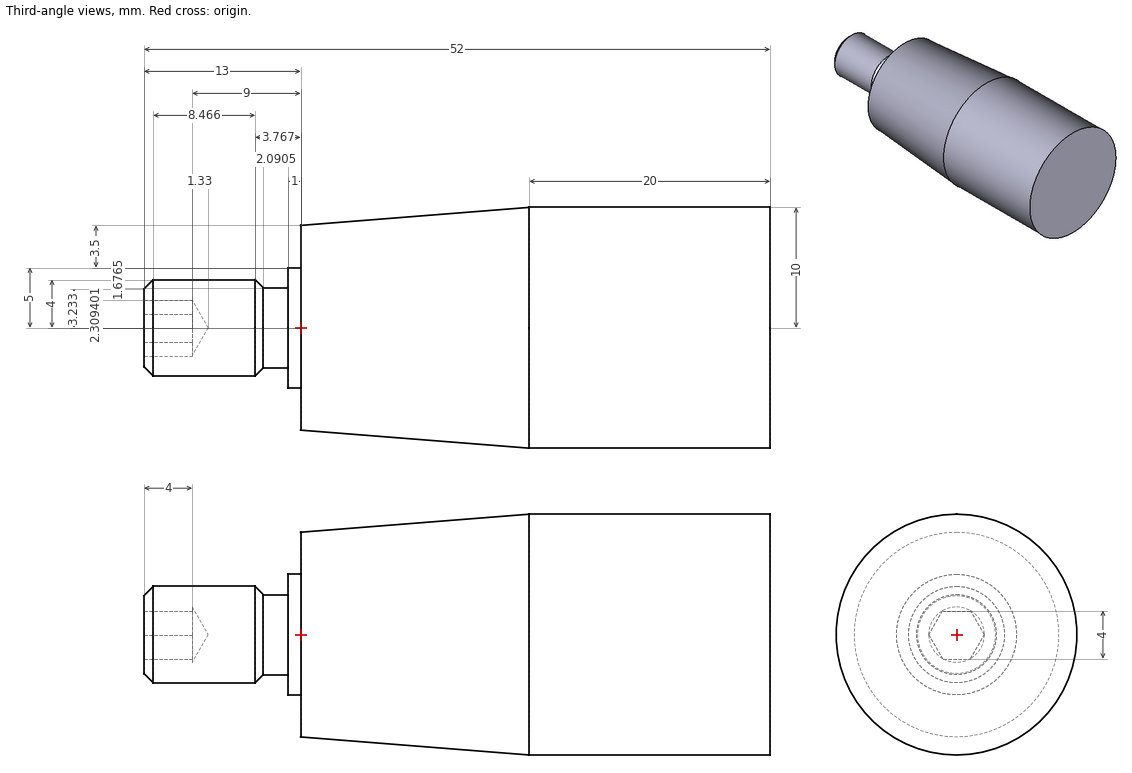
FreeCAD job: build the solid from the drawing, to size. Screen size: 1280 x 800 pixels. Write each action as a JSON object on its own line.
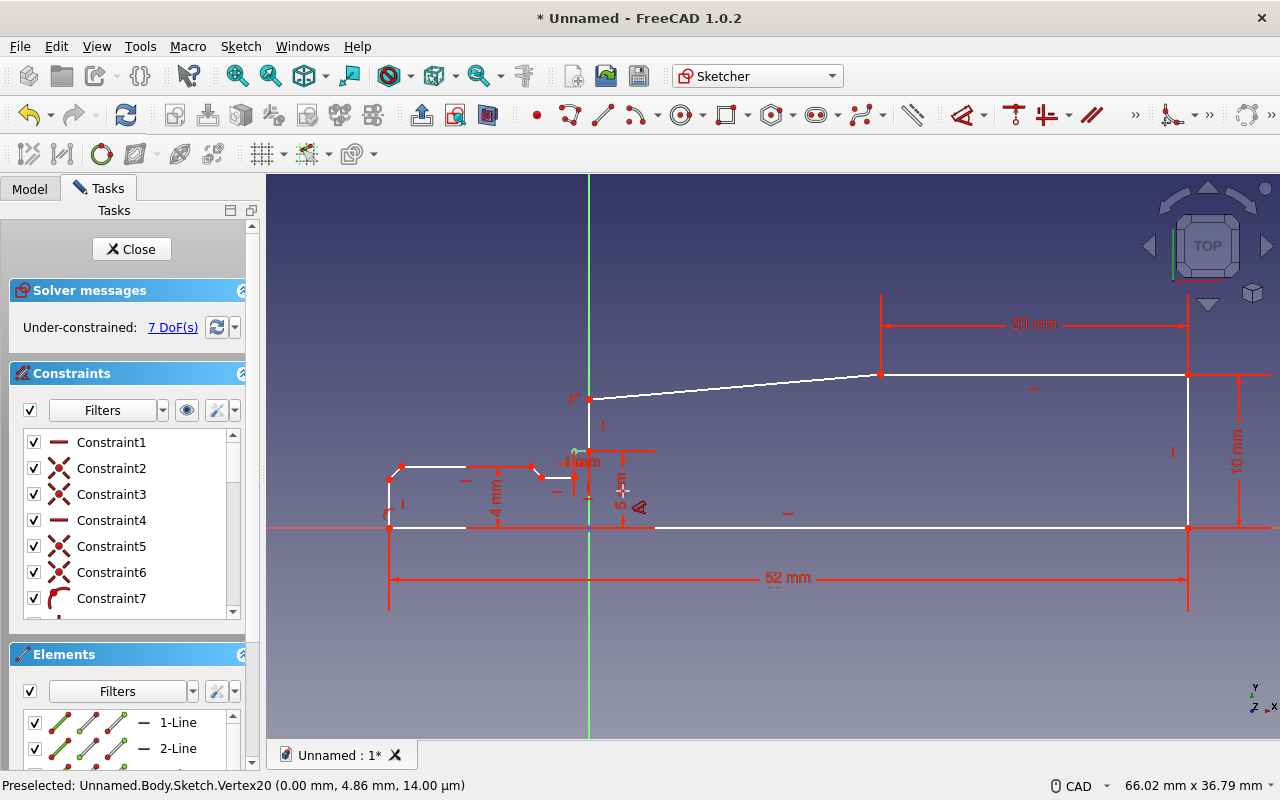
{"action": "left_click", "coordinate": [589, 415]}
{"action": "left_click", "coordinate": [555, 426]}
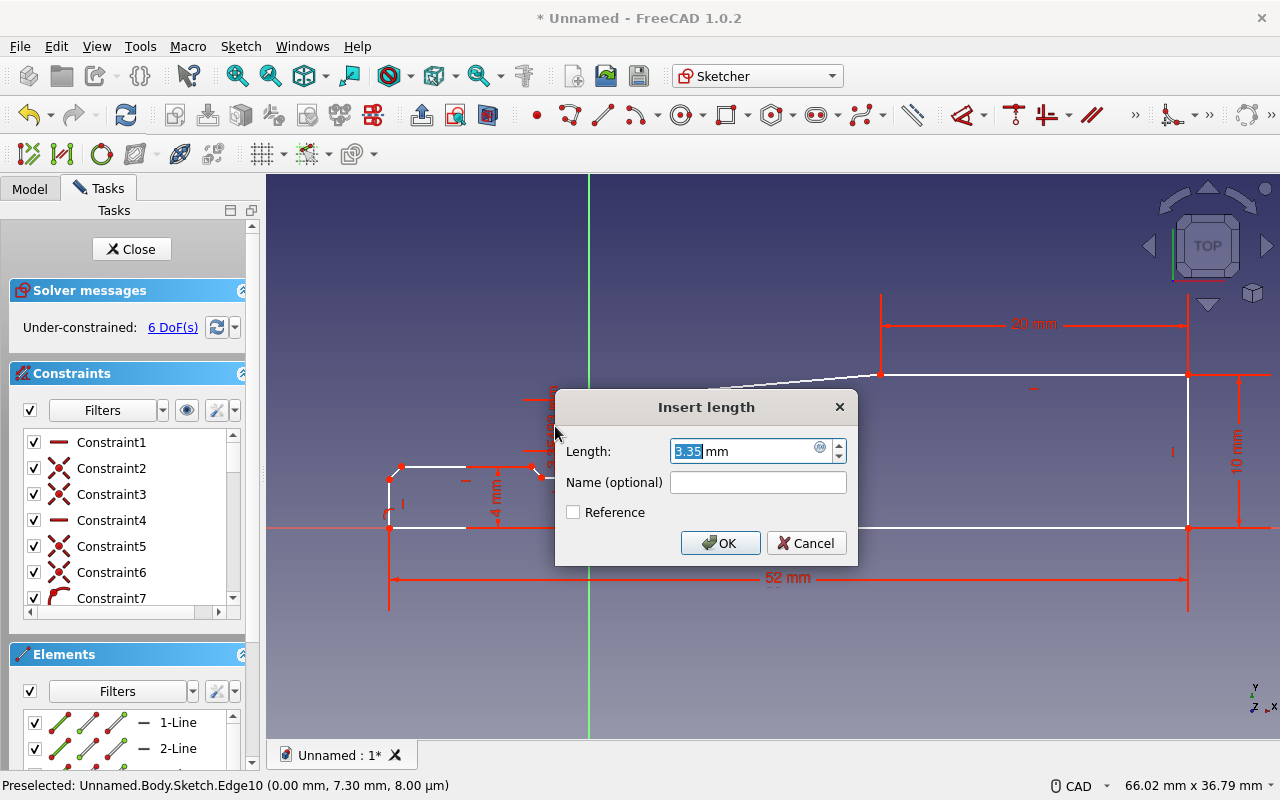
{"action": "type", "text": "3.5"}
{"action": "key", "text": "Return"}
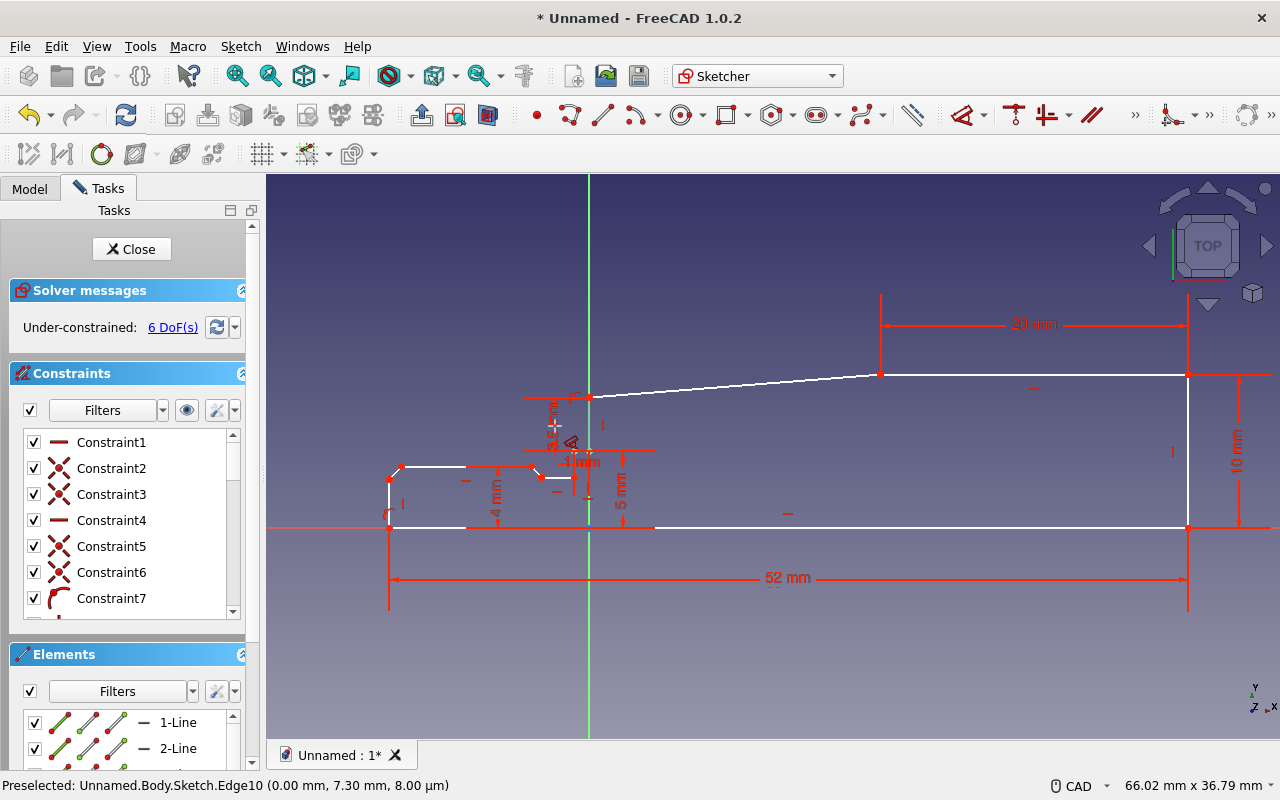
{"action": "left_click", "coordinate": [389, 479]}
{"action": "left_click", "coordinate": [489, 562]}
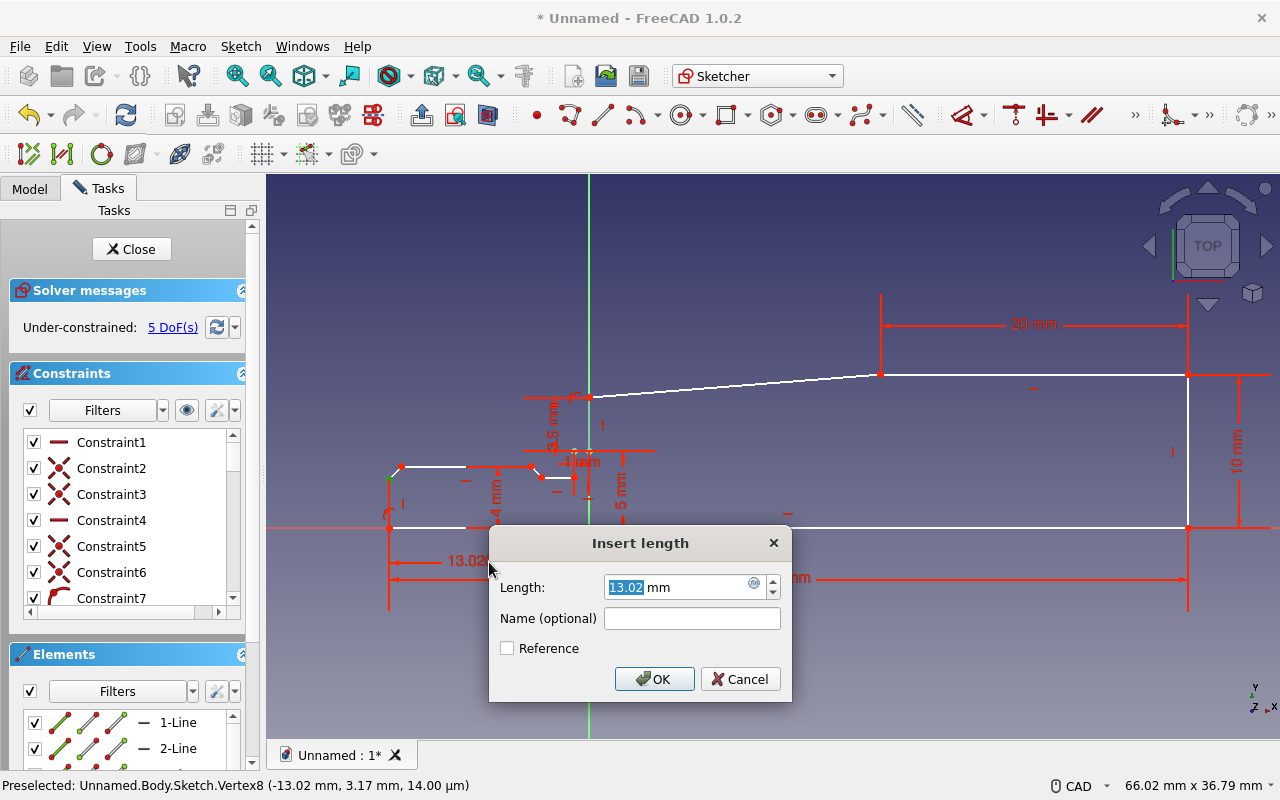
{"action": "type", "text": "13"}
{"action": "key", "text": "Return"}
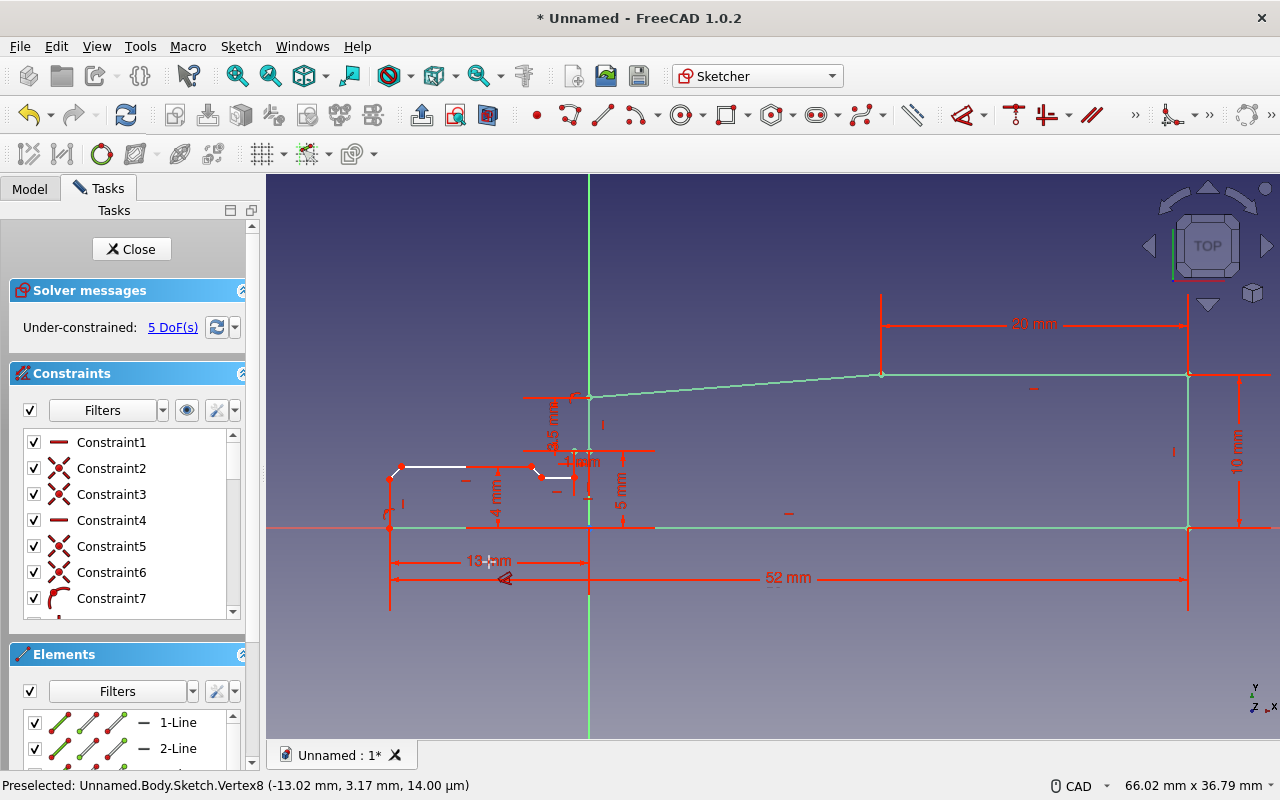
{"action": "left_click", "coordinate": [493, 467]}
{"action": "left_click", "coordinate": [421, 501]}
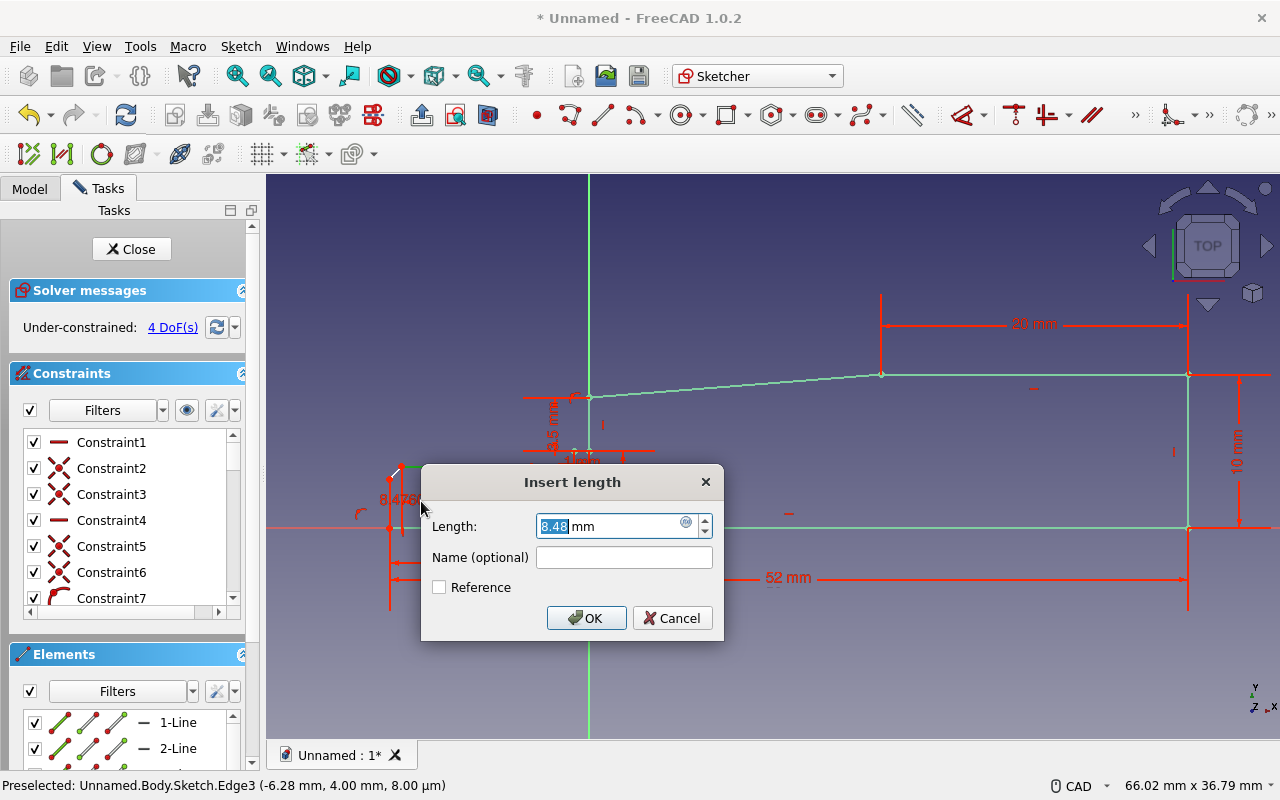
{"action": "type", "text": "8.466"}
{"action": "key", "text": "Return"}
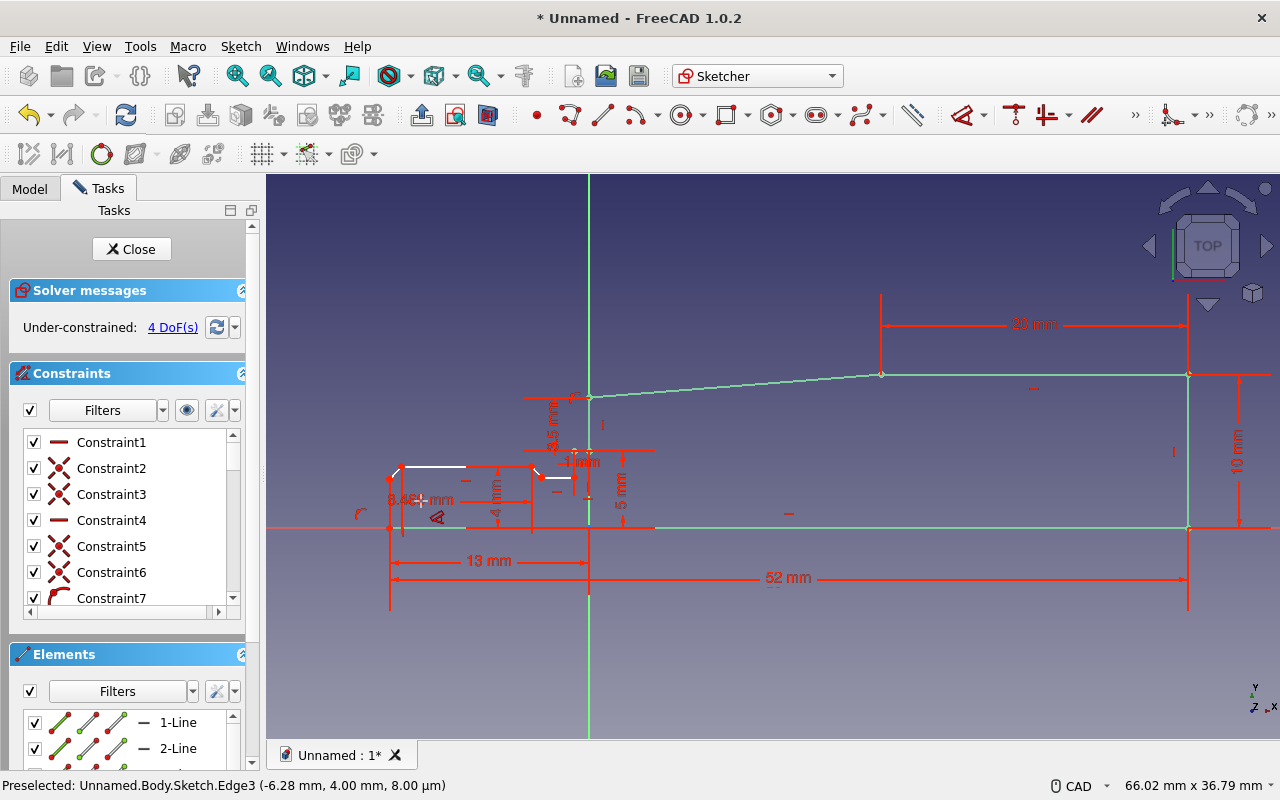
{"action": "left_click", "coordinate": [390, 494]}
{"action": "left_click", "coordinate": [332, 504]}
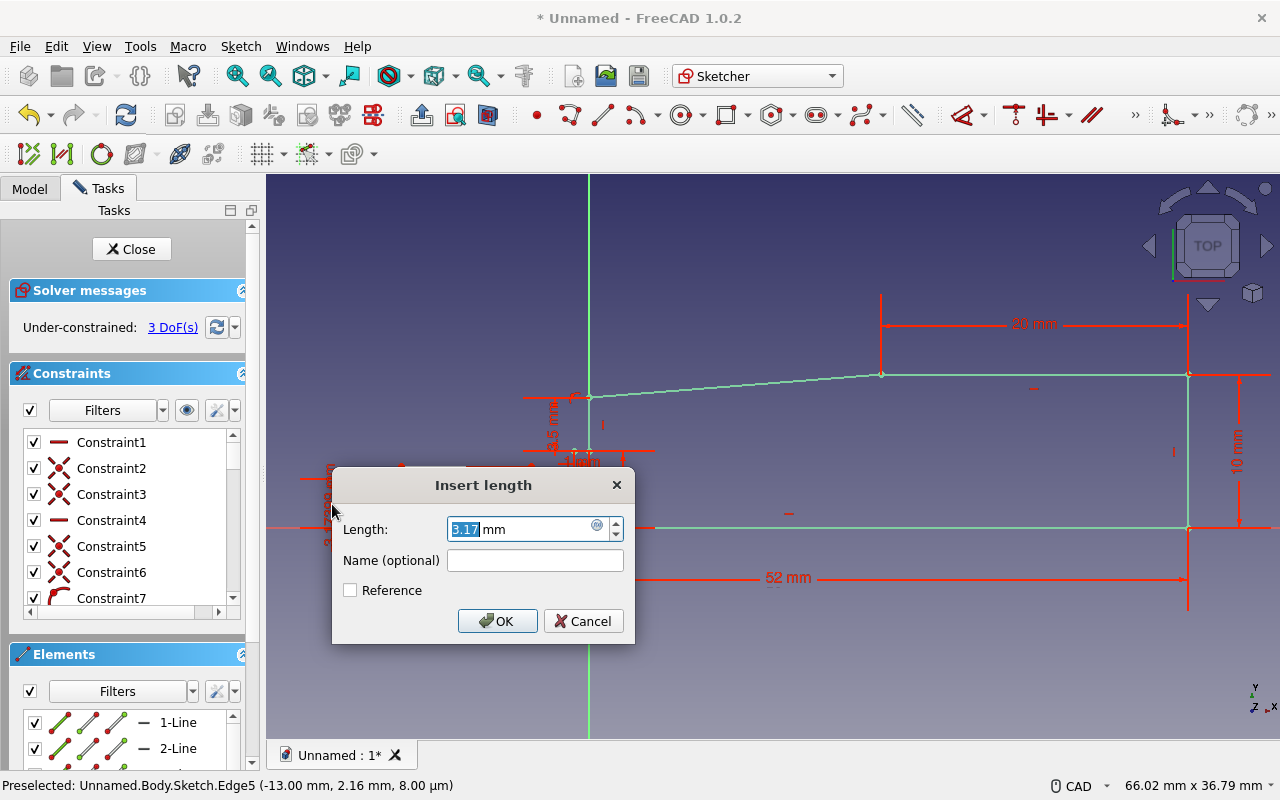
{"action": "type", "text": "3.233"}
{"action": "key", "text": "Return"}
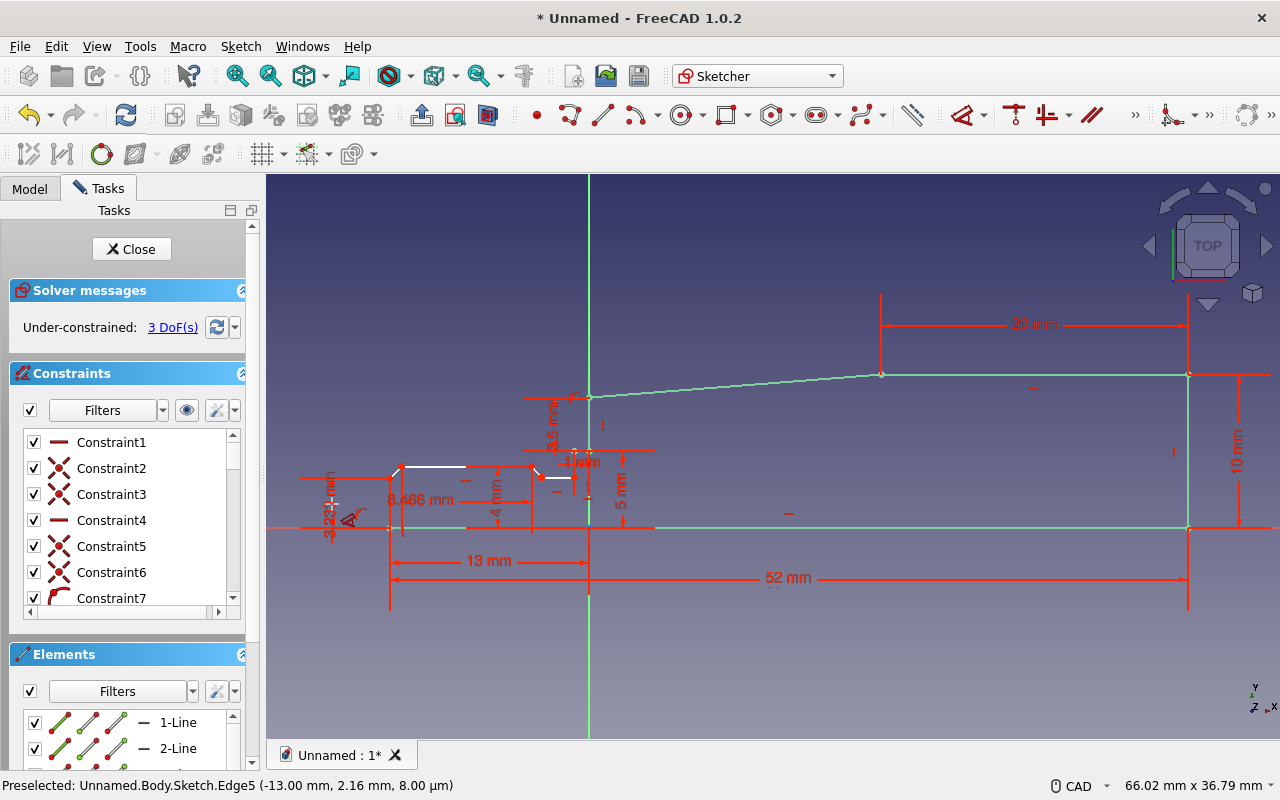
{"action": "scroll", "coordinate": [564, 478], "scroll_direction": "up", "scroll_amount": 2}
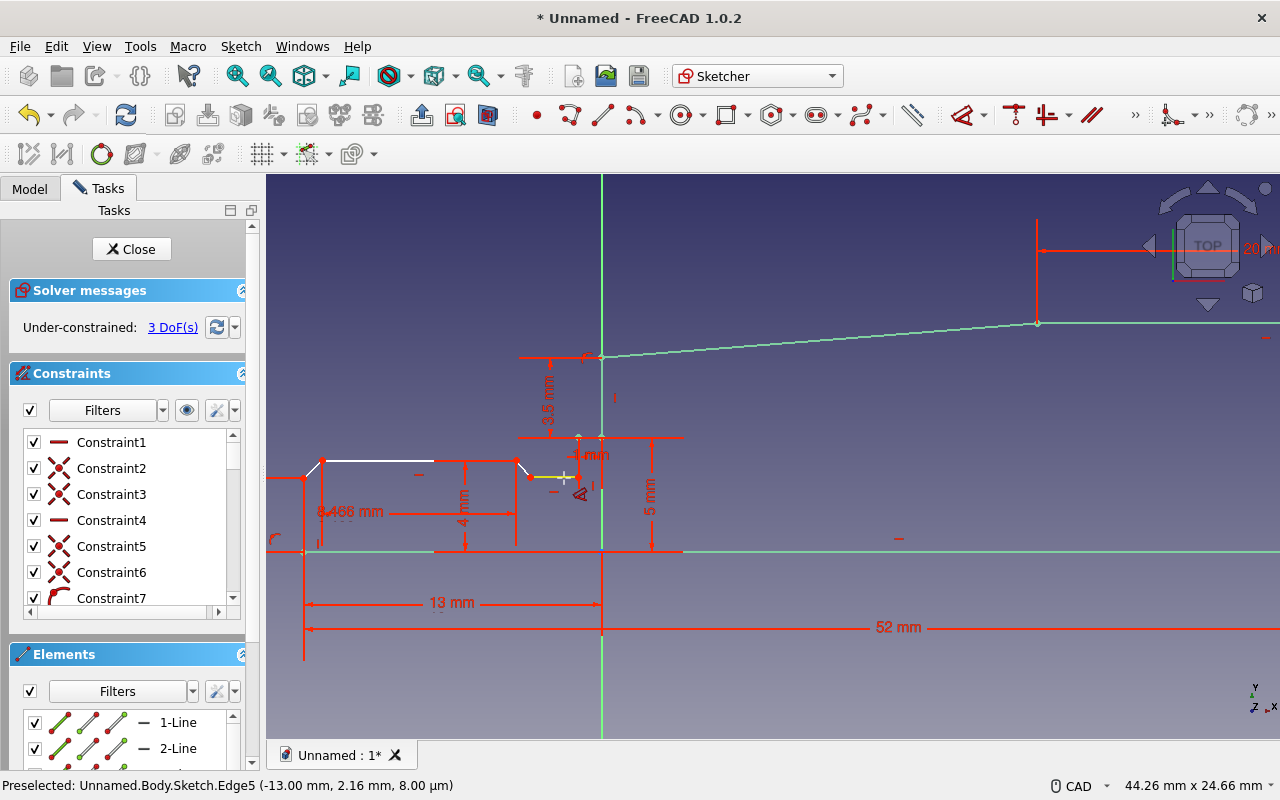
{"action": "left_click", "coordinate": [564, 477]}
{"action": "left_click", "coordinate": [555, 511]}